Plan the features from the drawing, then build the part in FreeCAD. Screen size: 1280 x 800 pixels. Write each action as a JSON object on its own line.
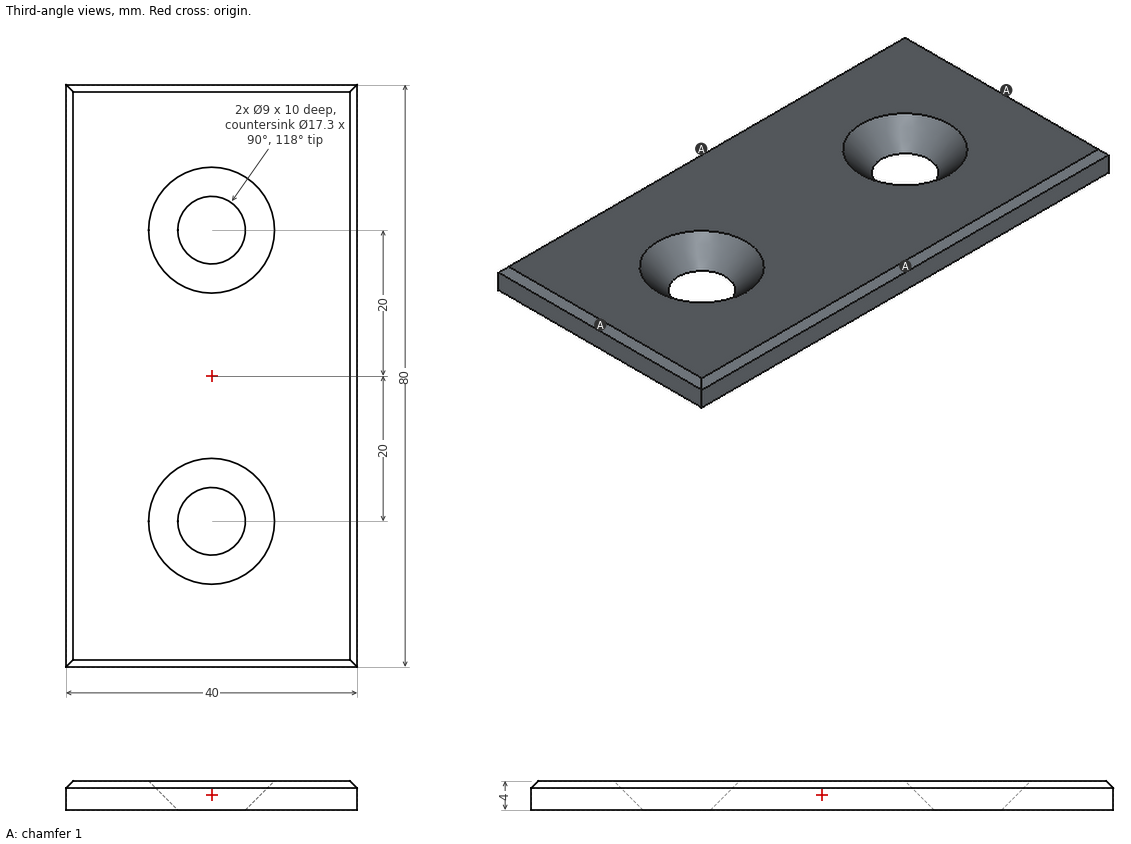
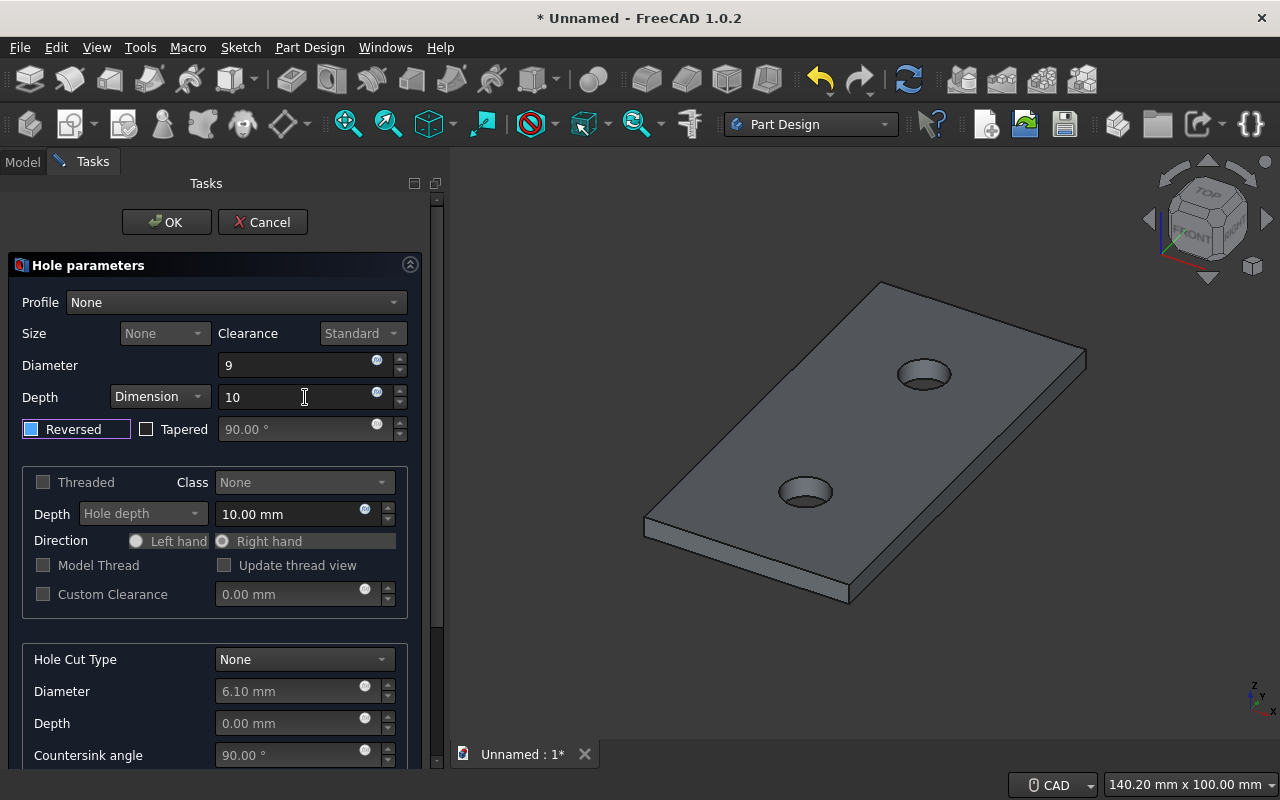
{"action": "left_click", "coordinate": [306, 660]}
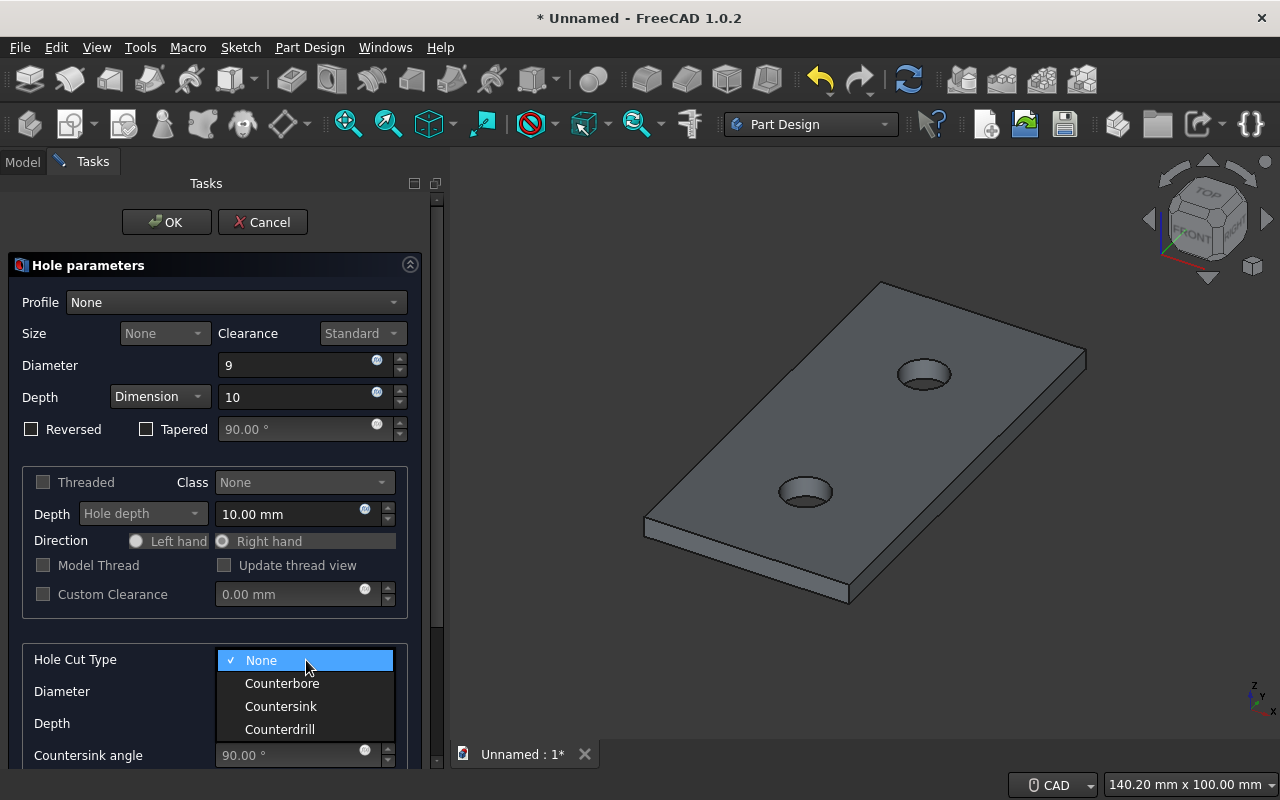
{"action": "left_click", "coordinate": [304, 706]}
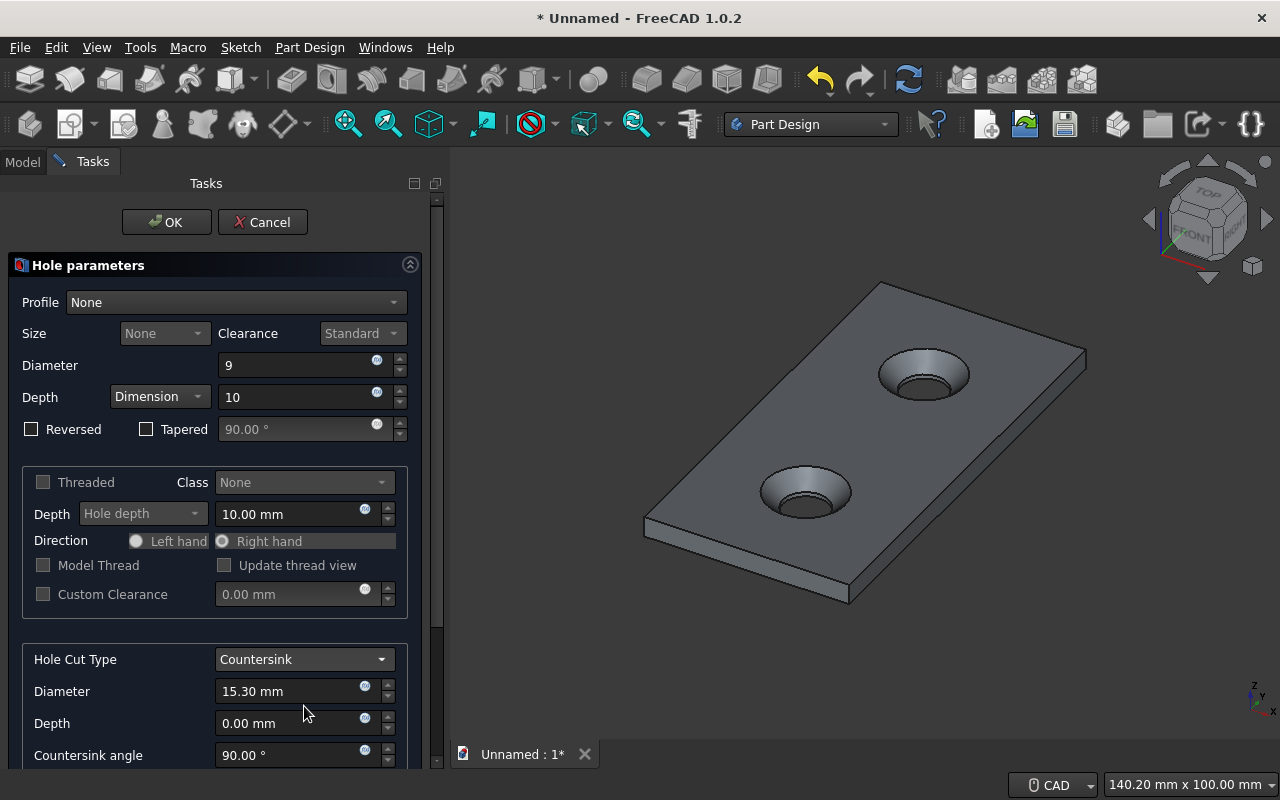
{"action": "triple_click", "coordinate": [298, 691]}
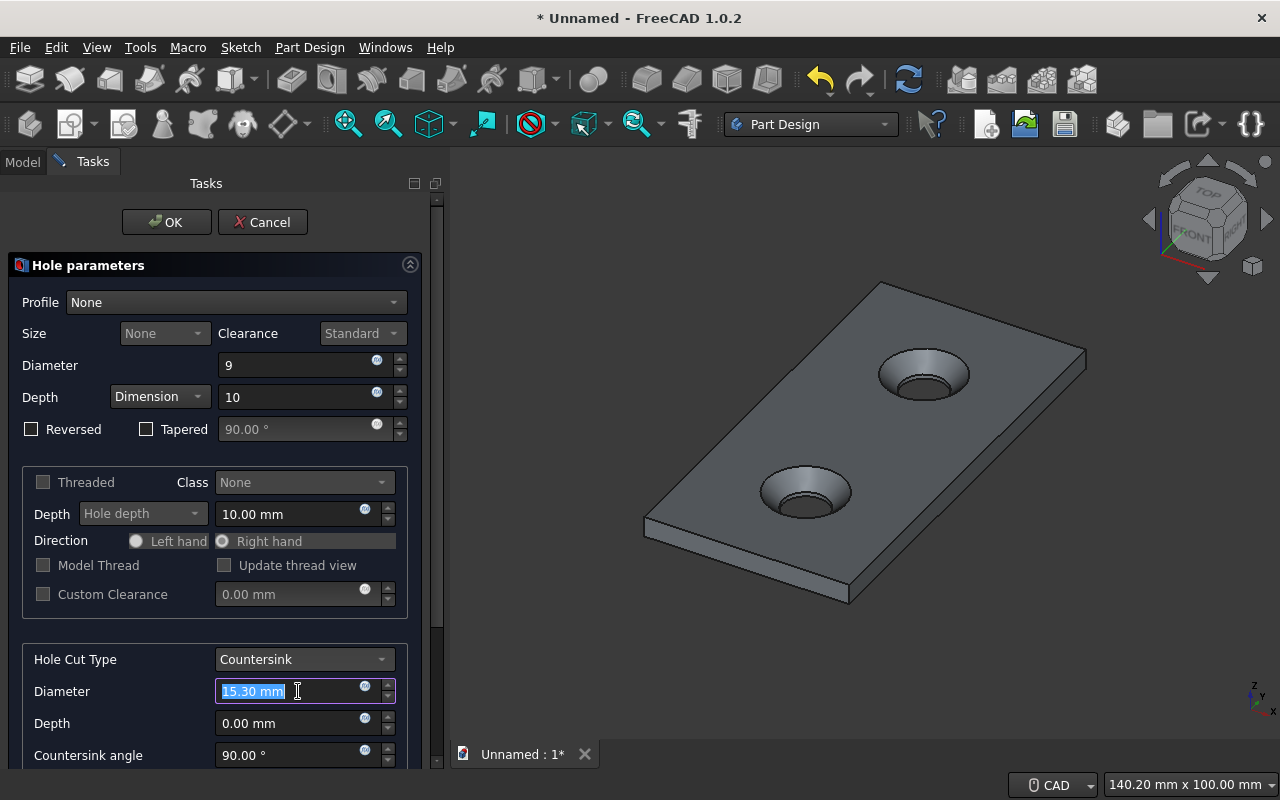
{"action": "type", "text": "17.3"}
{"action": "key", "text": "Tab"}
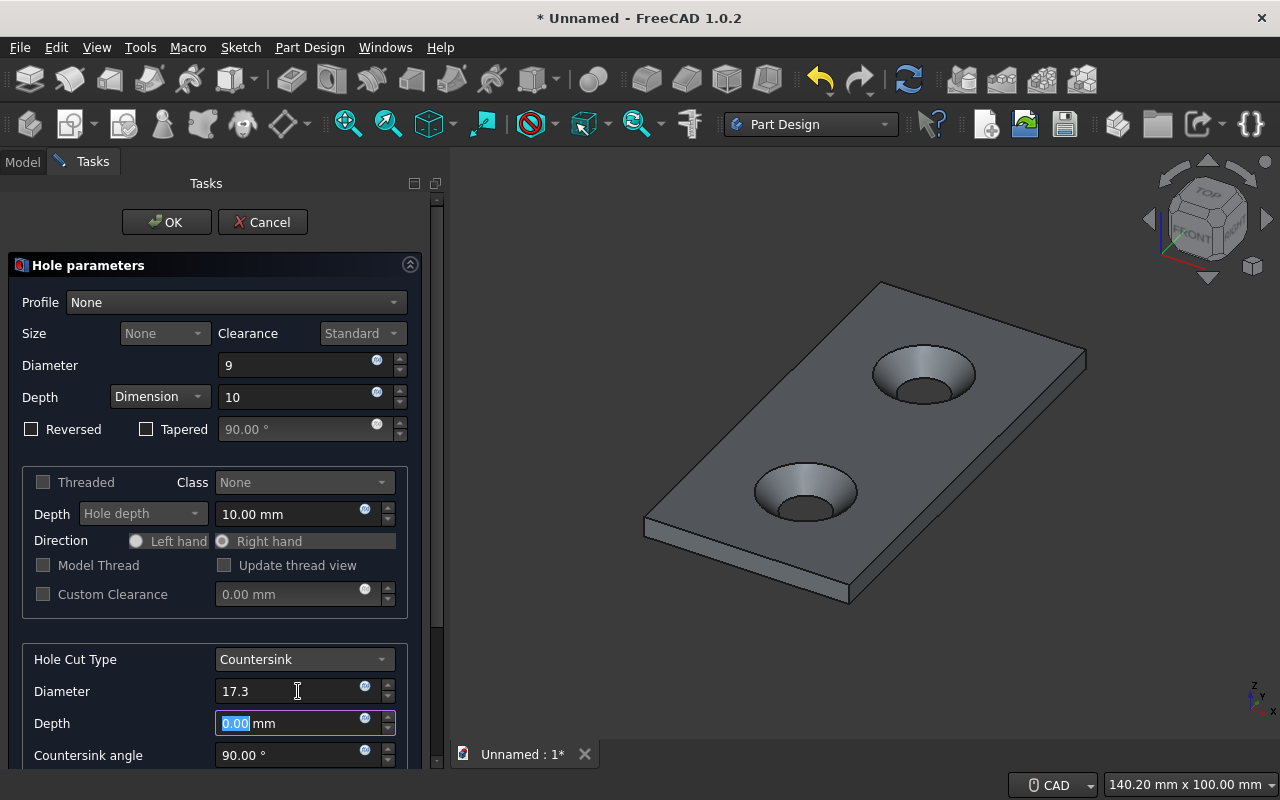
{"action": "left_click", "coordinate": [167, 222]}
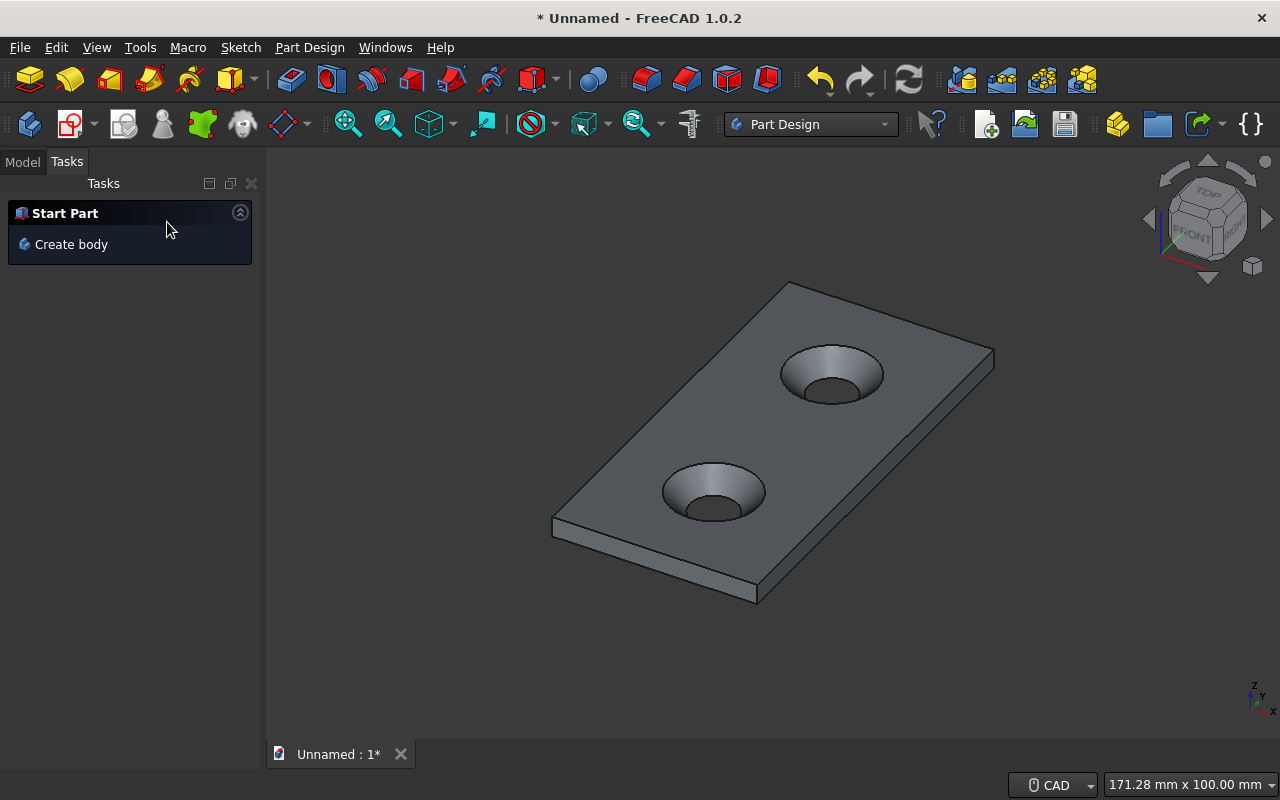
{"action": "left_click", "coordinate": [655, 550]}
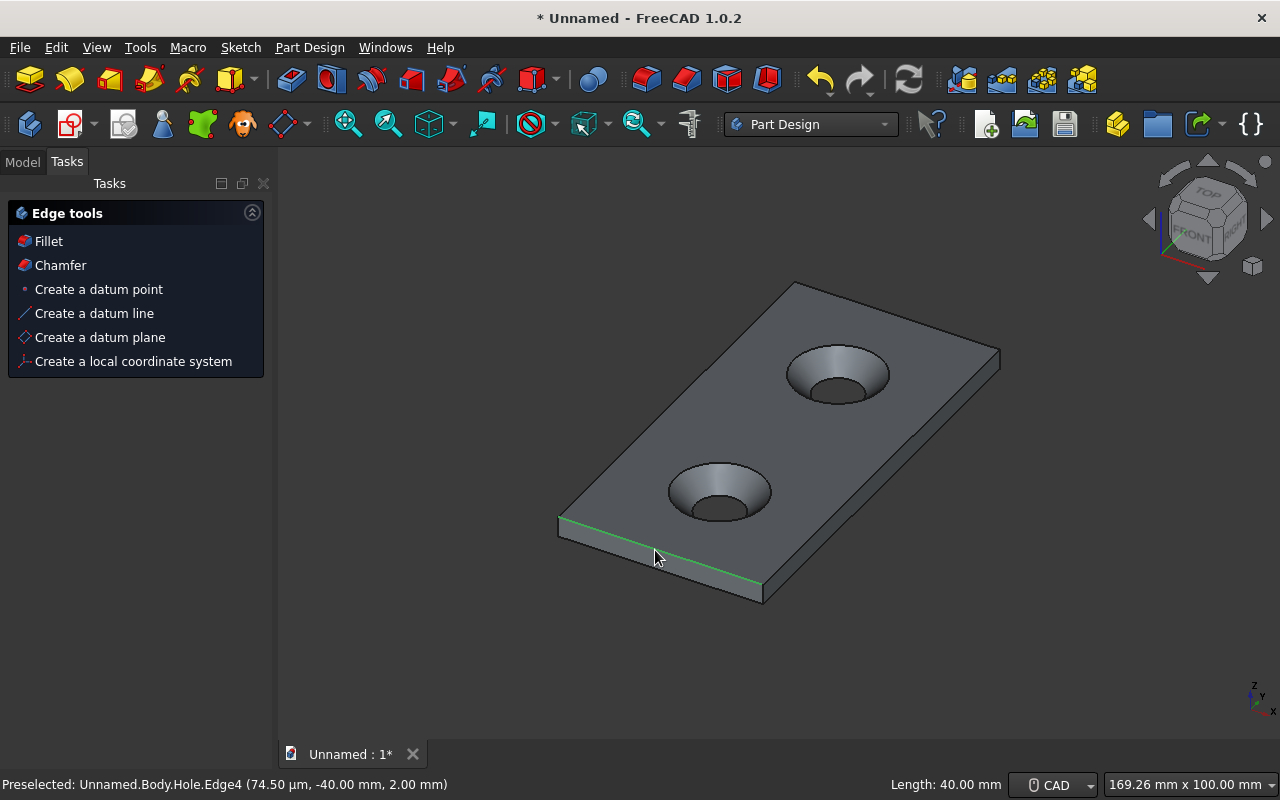
{"action": "left_click", "coordinate": [882, 466], "text": "ctrl"}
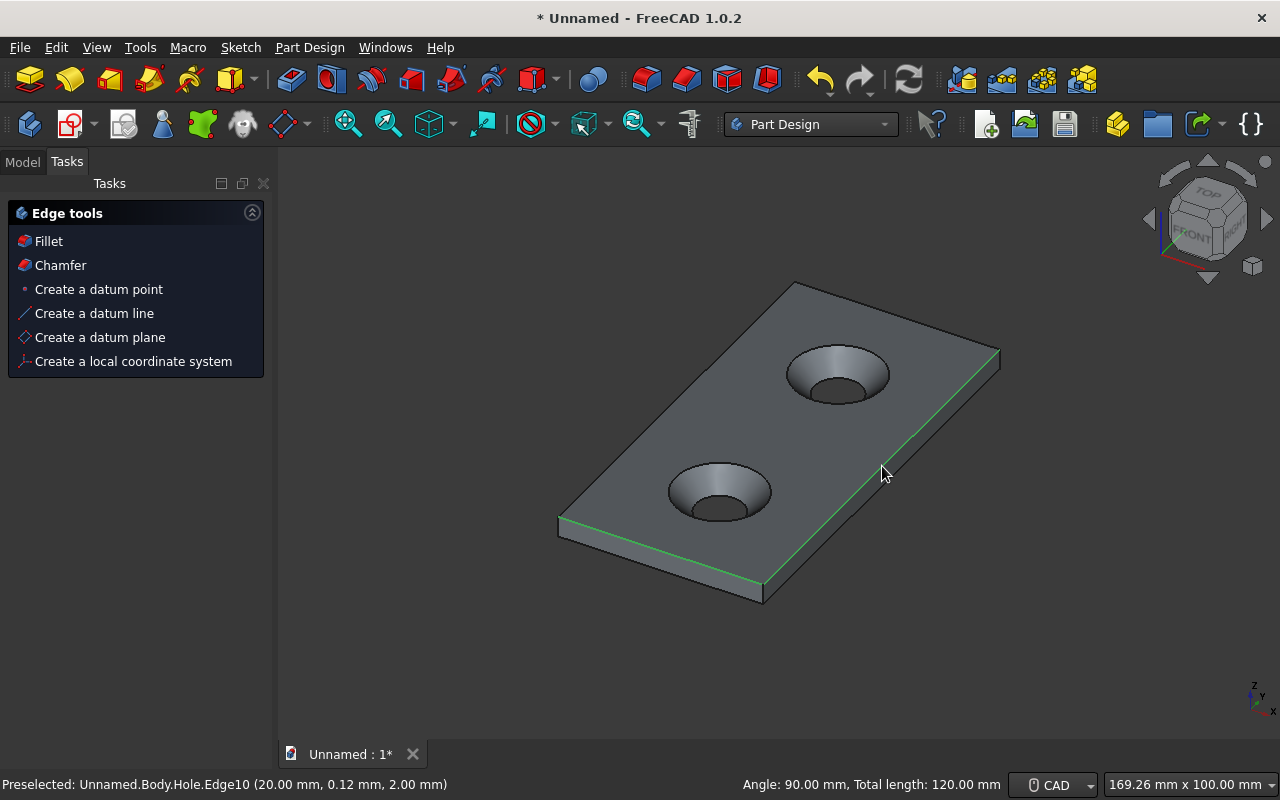
{"action": "key", "text": "0"}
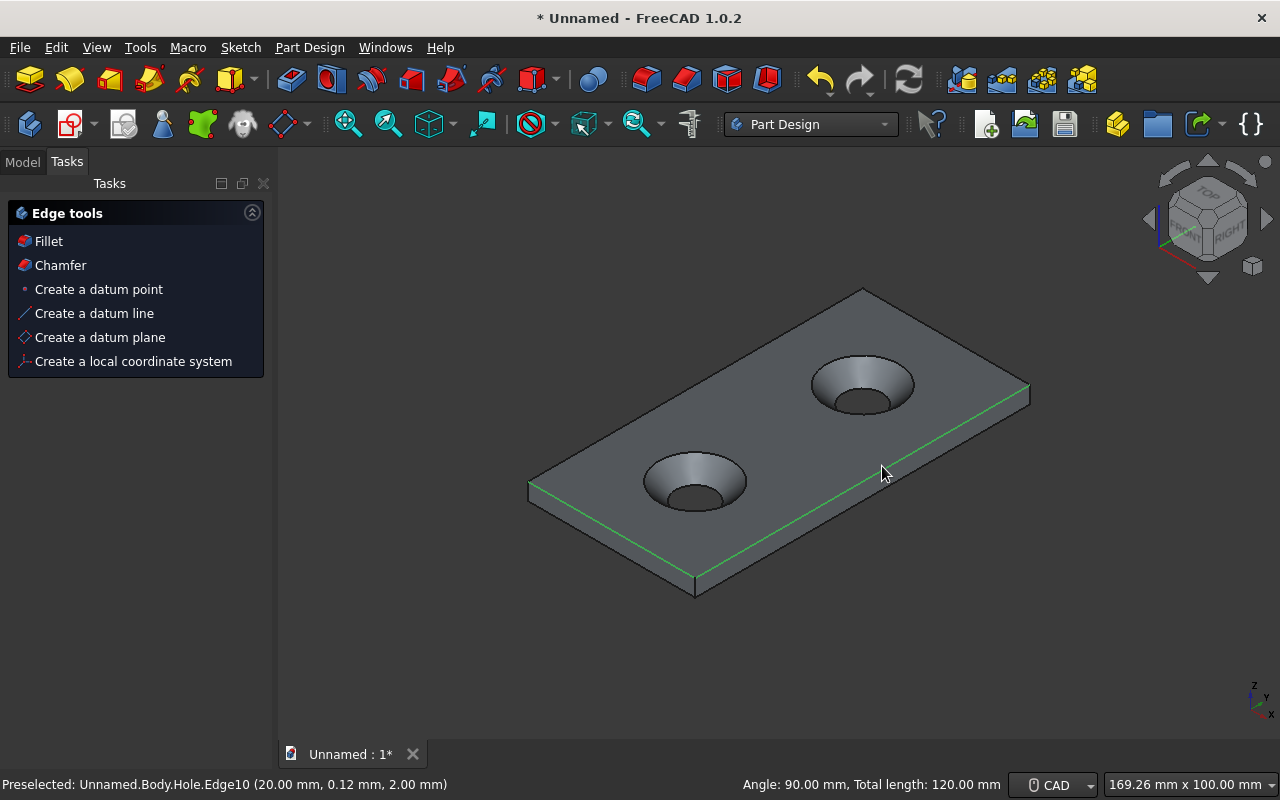
{"action": "key", "text": "2"}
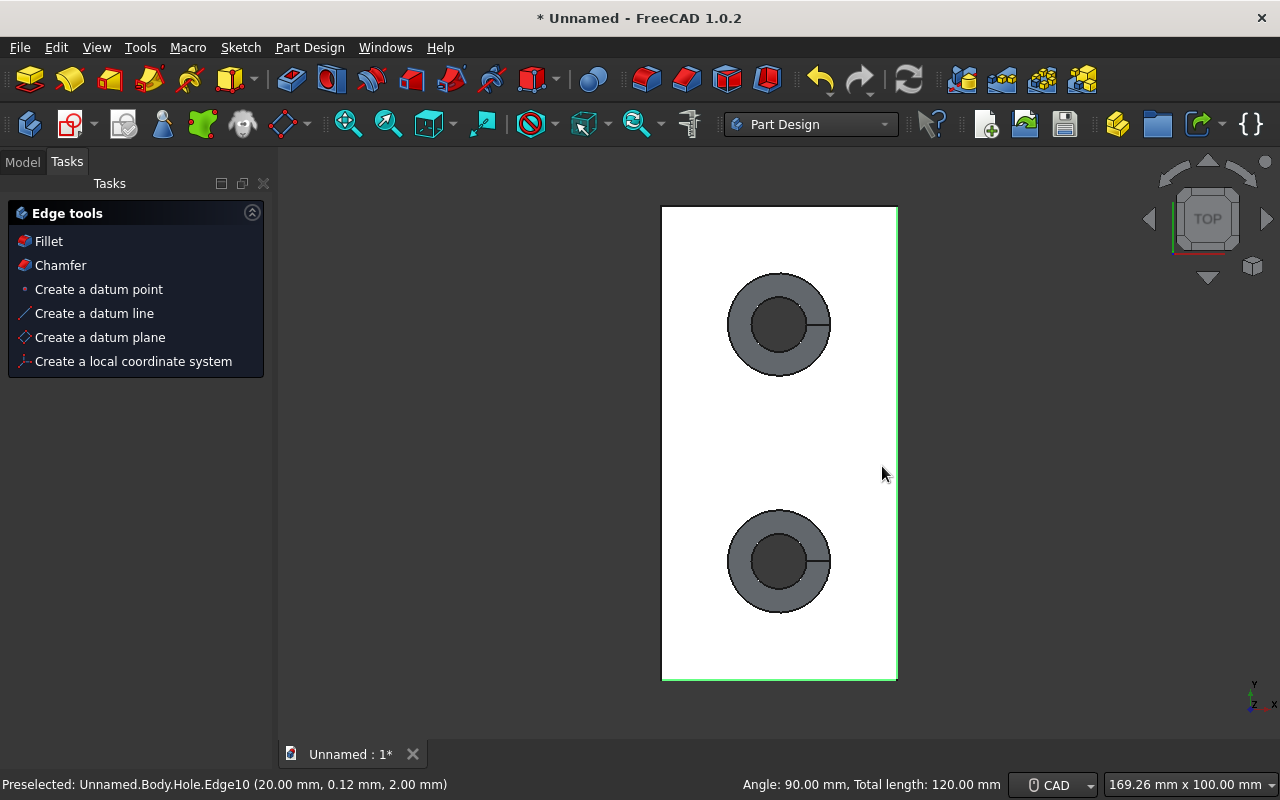
{"action": "left_click", "coordinate": [661, 442], "text": "ctrl"}